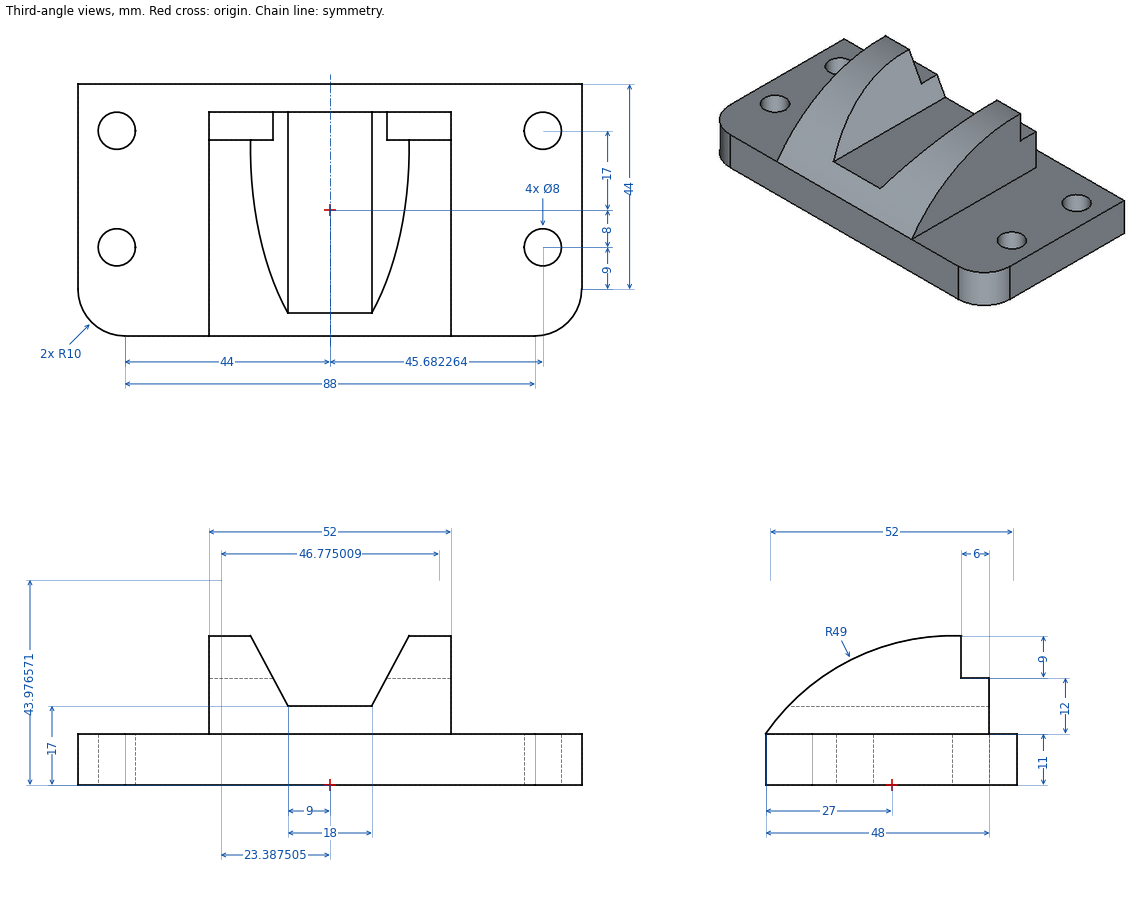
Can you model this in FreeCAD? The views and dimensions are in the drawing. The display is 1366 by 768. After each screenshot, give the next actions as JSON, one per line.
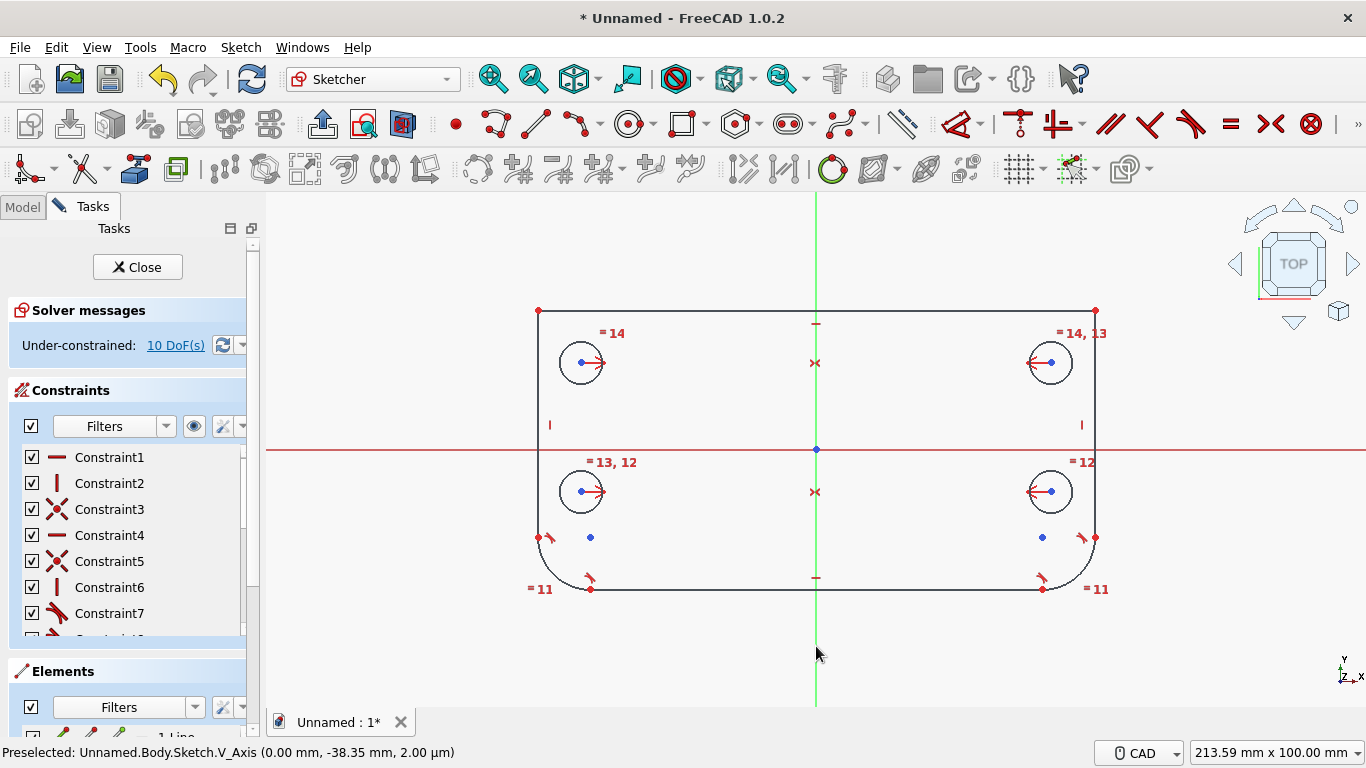
{"action": "left_click", "coordinate": [1066, 584]}
{"action": "left_click", "coordinate": [1080, 613]}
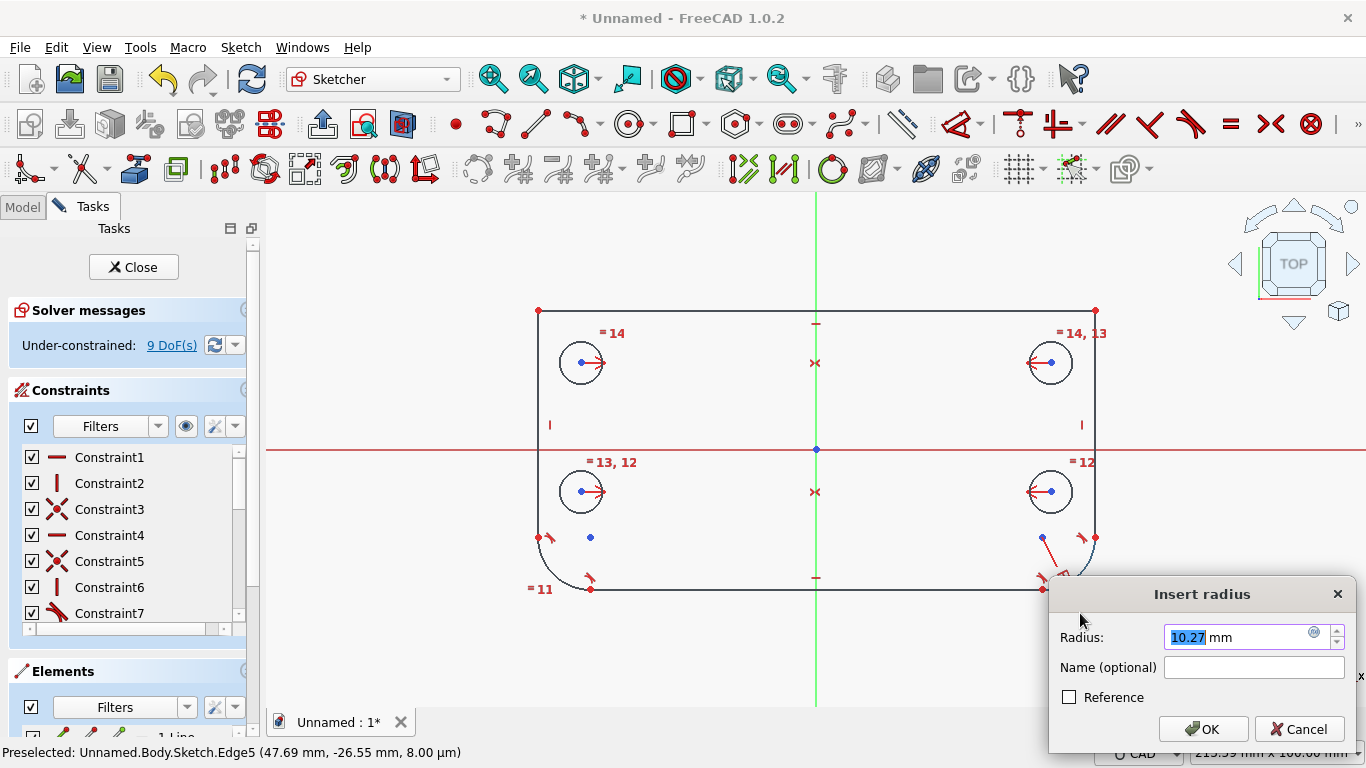
{"action": "type", "text": "10"}
{"action": "key", "text": "Return"}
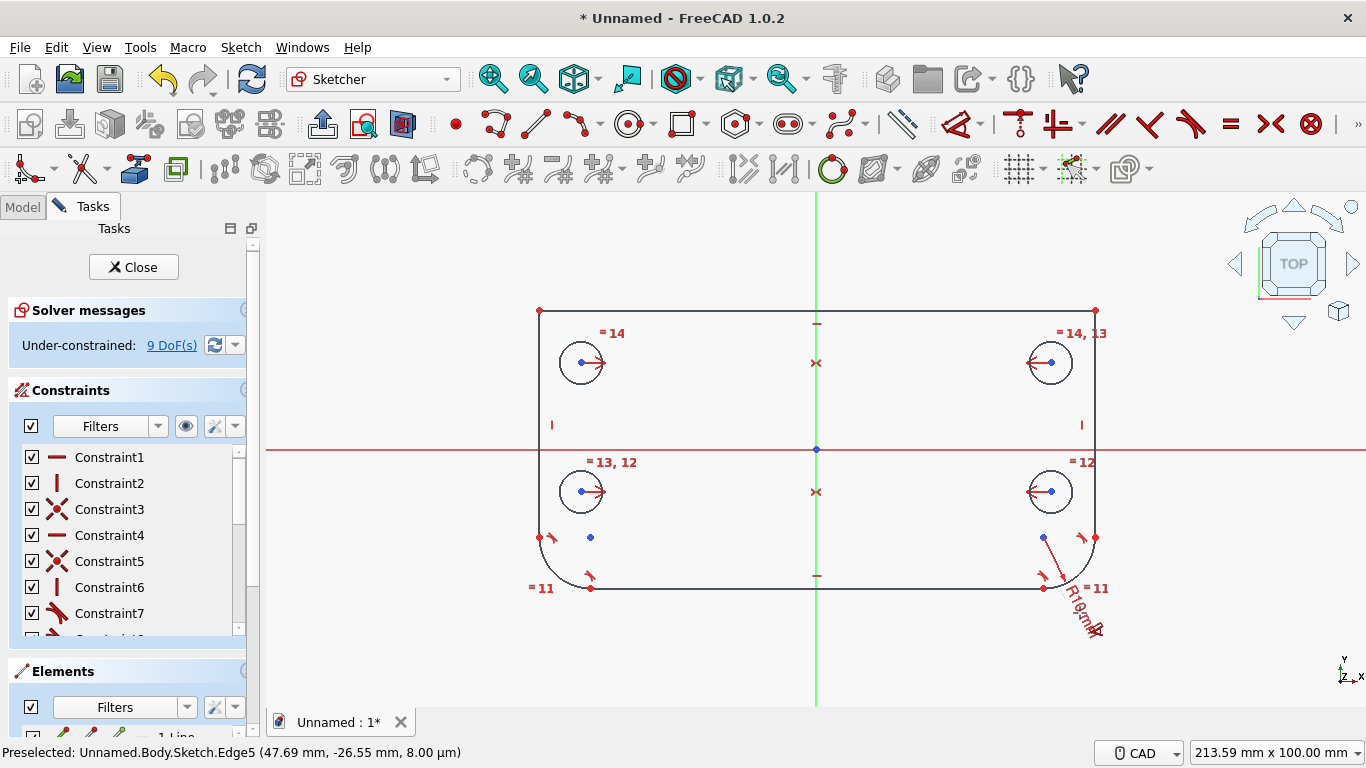
{"action": "left_click", "coordinate": [1066, 477]}
{"action": "left_click", "coordinate": [1013, 530]}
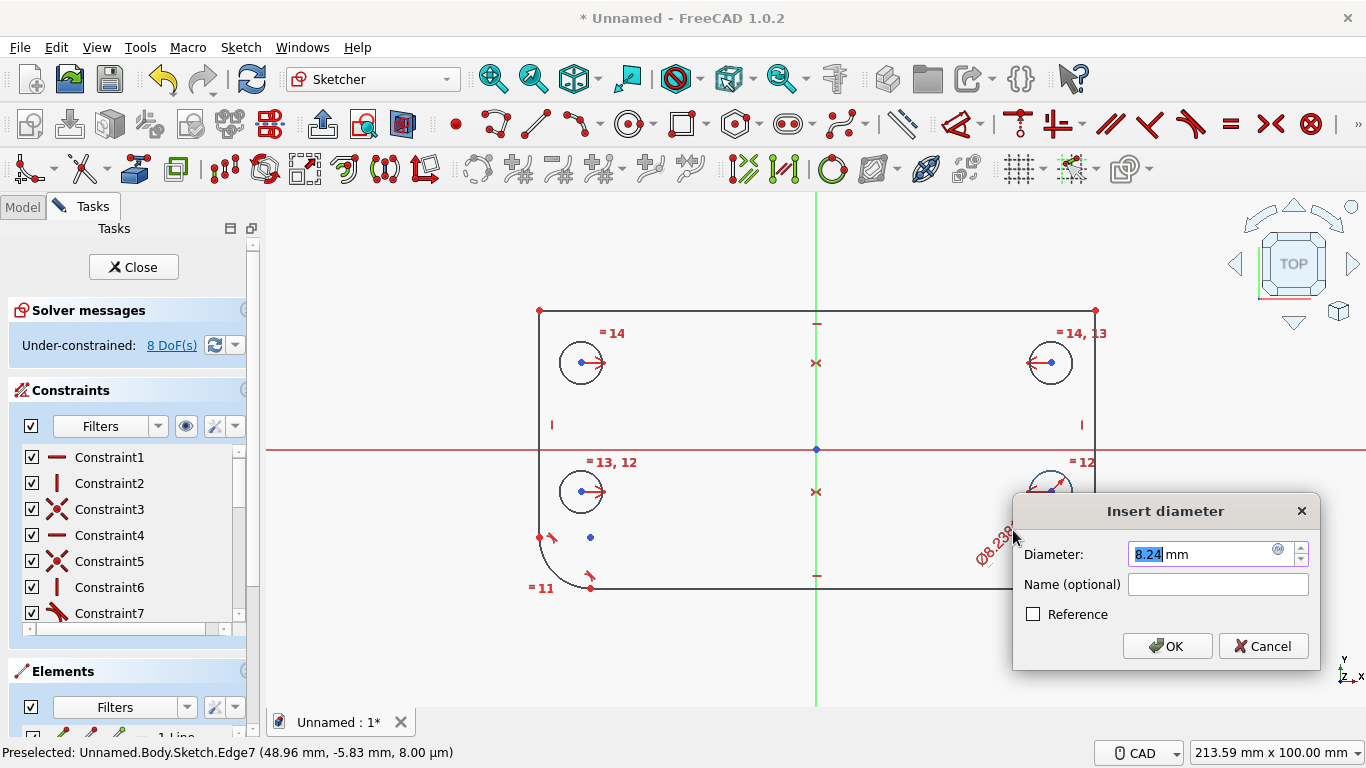
{"action": "type", "text": "8"}
{"action": "key", "text": "Return"}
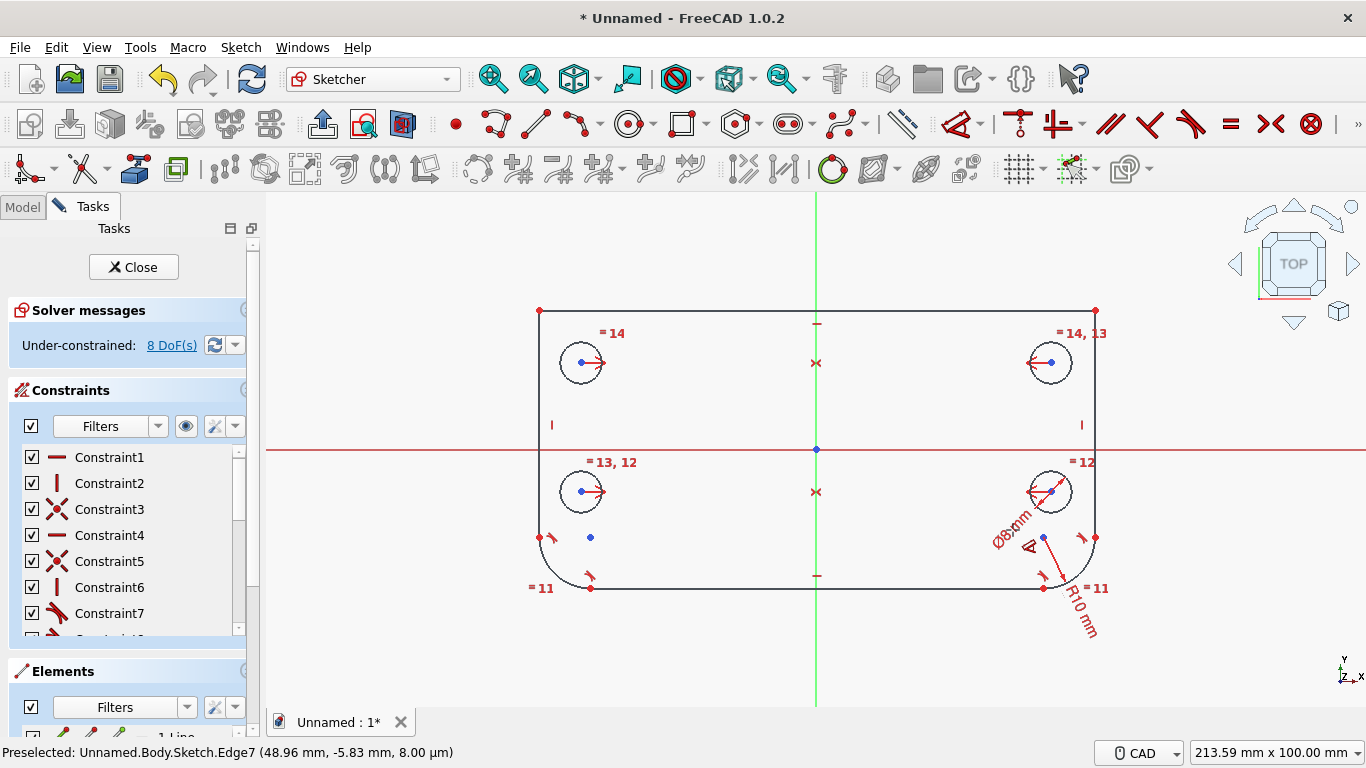
{"action": "left_click", "coordinate": [1051, 492]}
{"action": "left_click", "coordinate": [782, 471]}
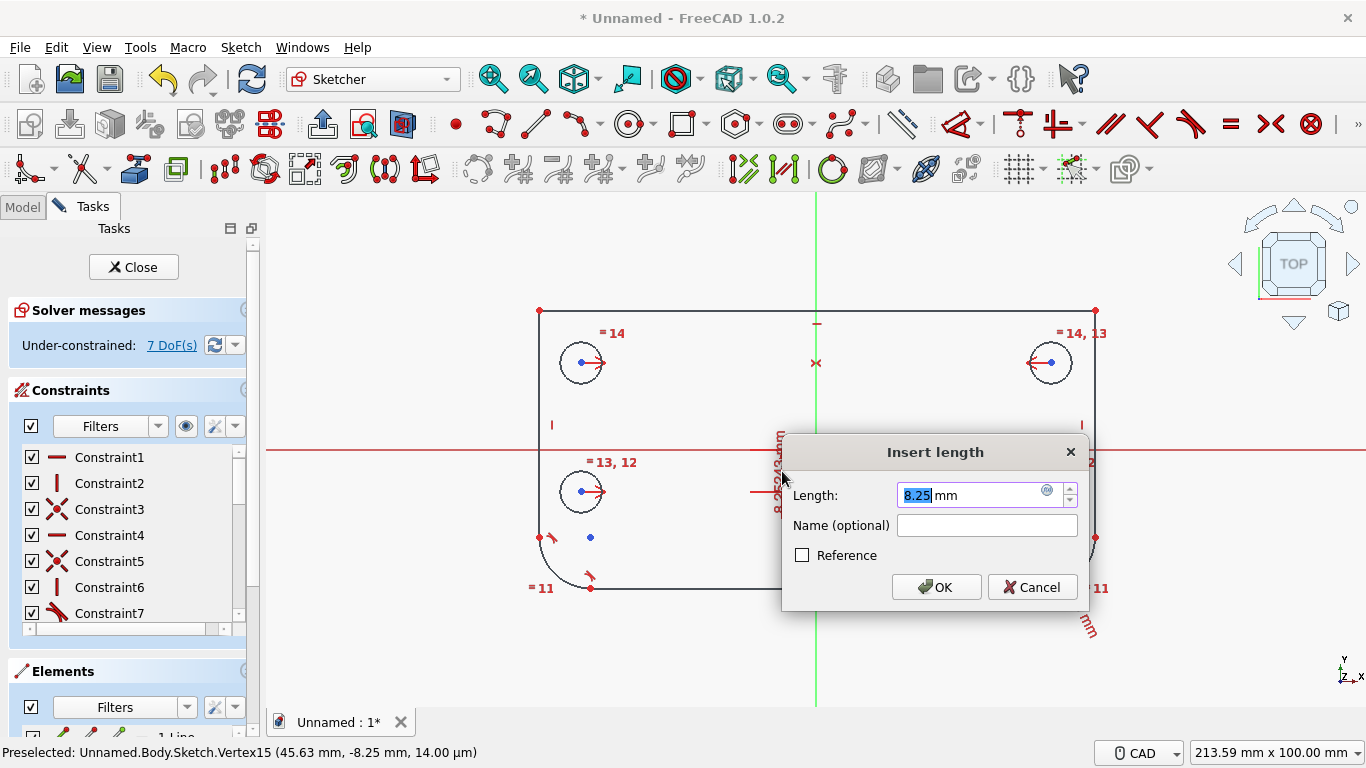
{"action": "type", "text": "8"}
{"action": "key", "text": "Return"}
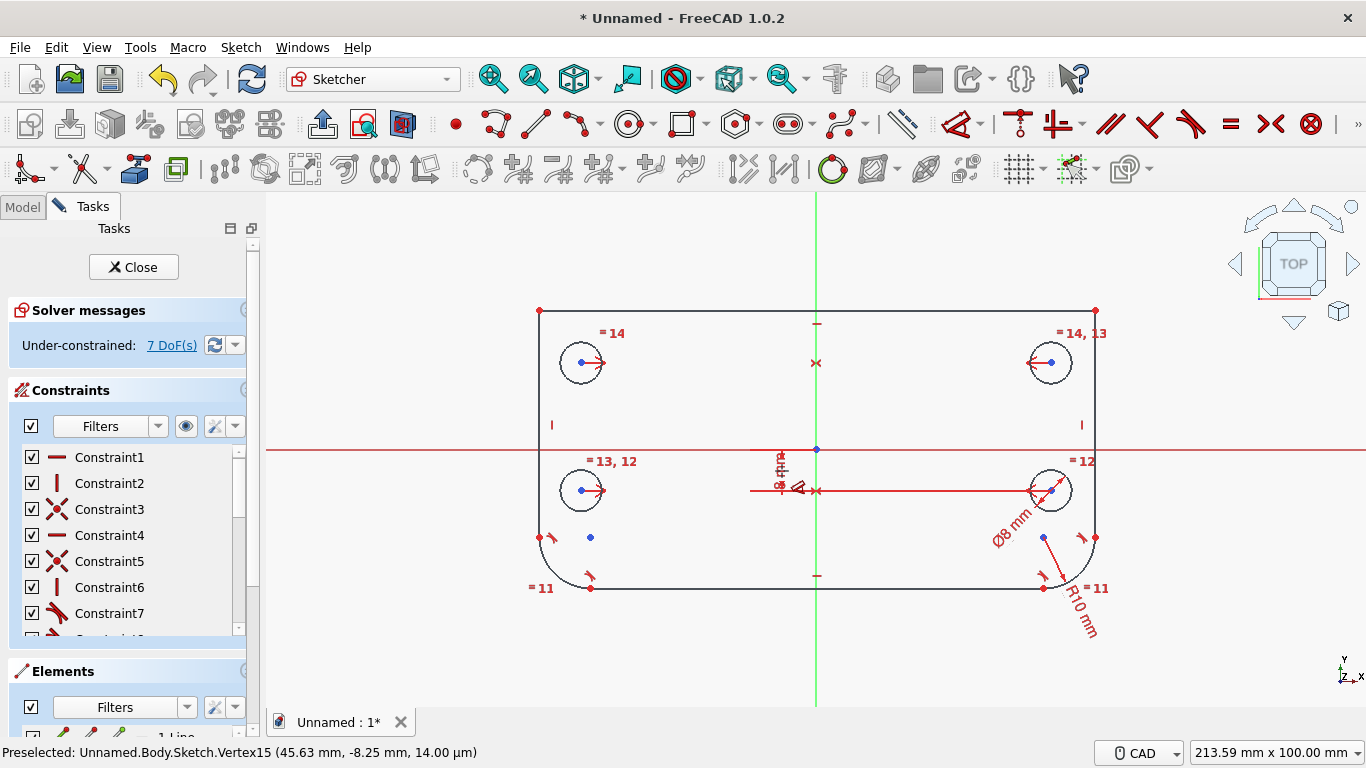
{"action": "left_click", "coordinate": [727, 589]}
{"action": "left_click", "coordinate": [713, 623]}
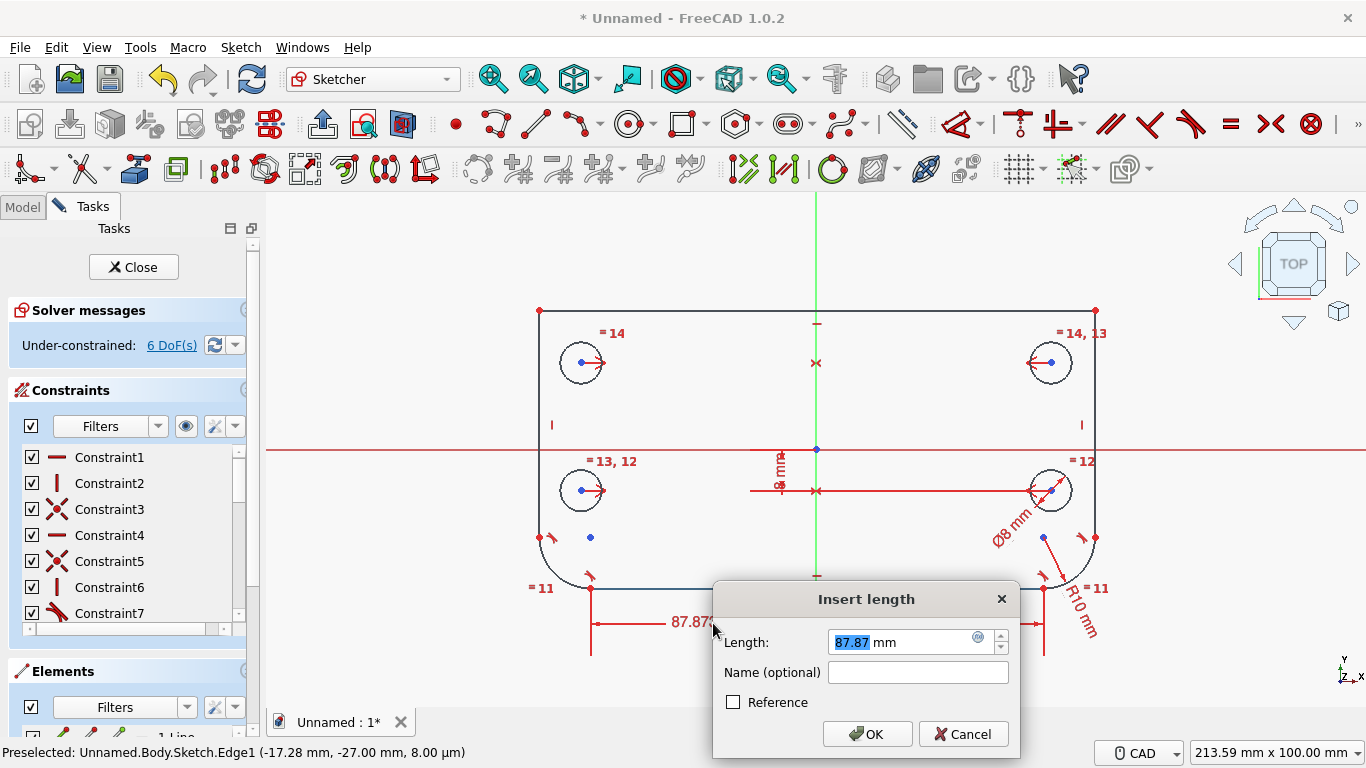
{"action": "type", "text": "88"}
{"action": "key", "text": "Return"}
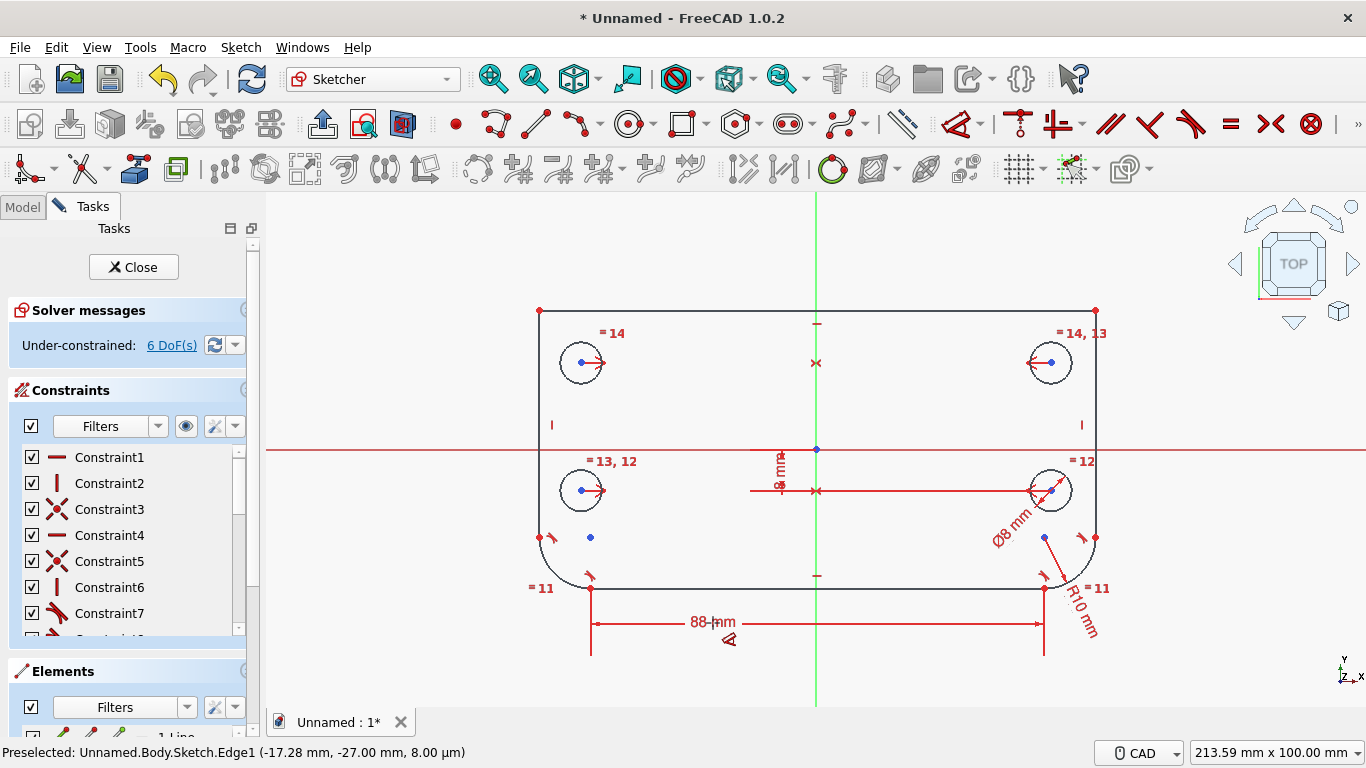
{"action": "left_click", "coordinate": [1096, 469]}
{"action": "left_click", "coordinate": [1130, 424]}